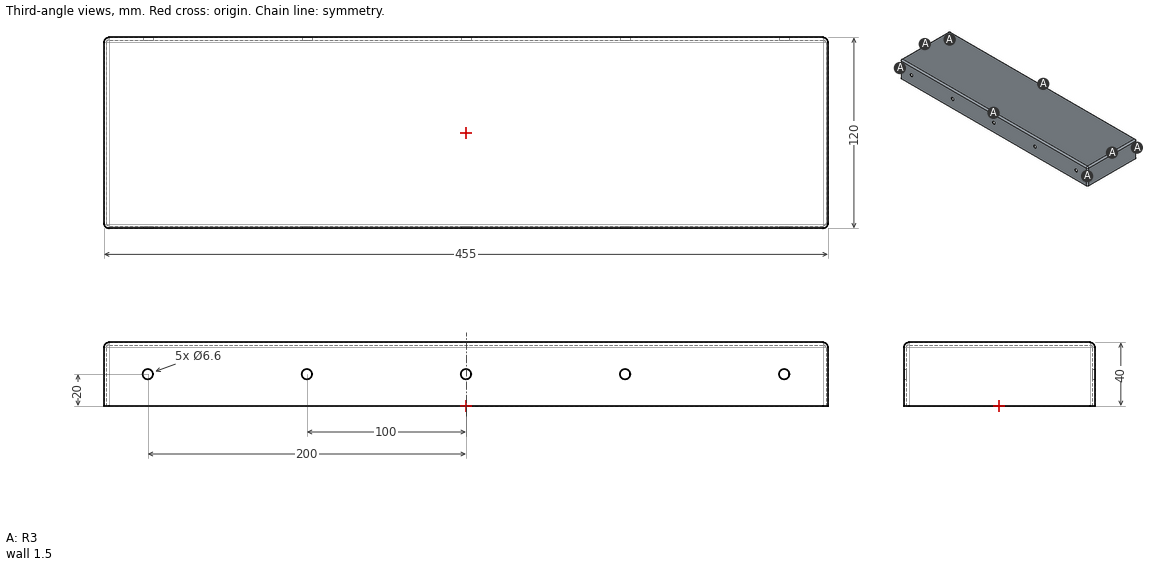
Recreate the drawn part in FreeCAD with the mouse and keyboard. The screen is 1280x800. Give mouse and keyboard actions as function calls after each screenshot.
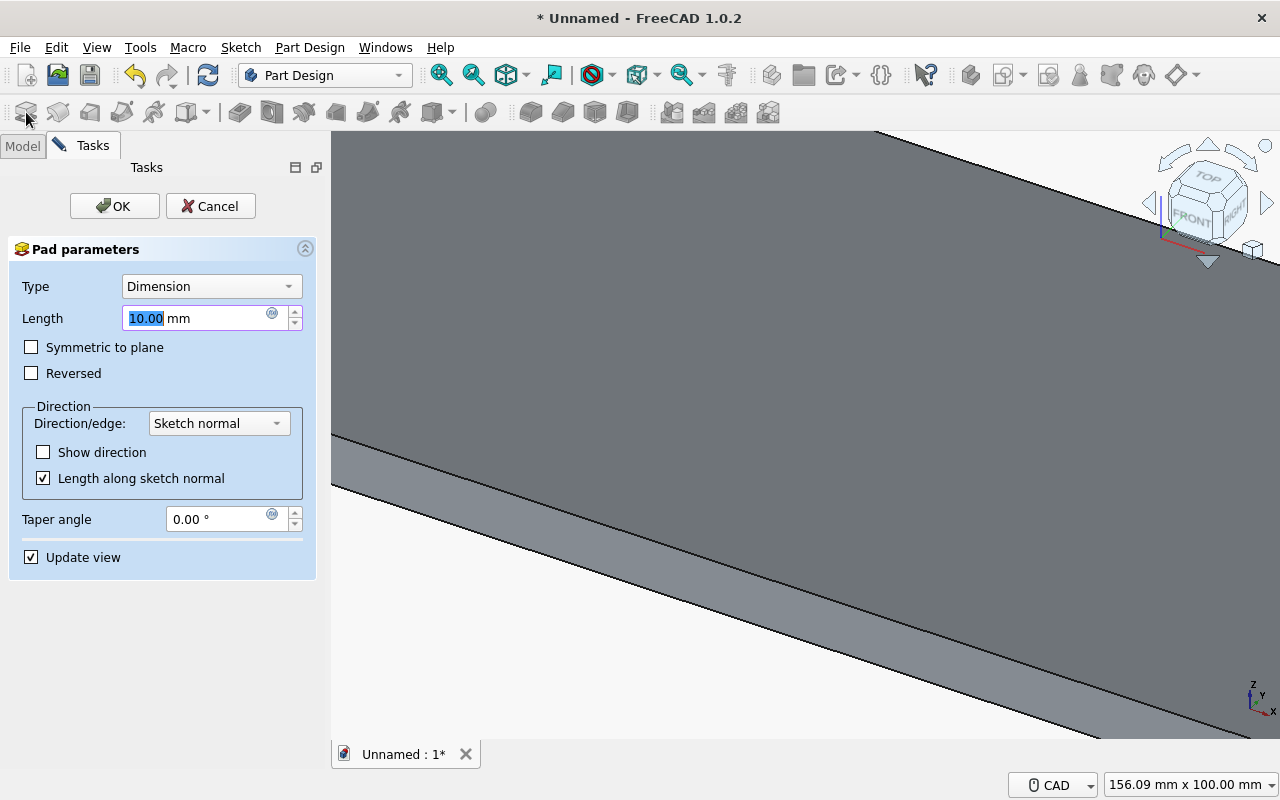
text(40)
key(Tab)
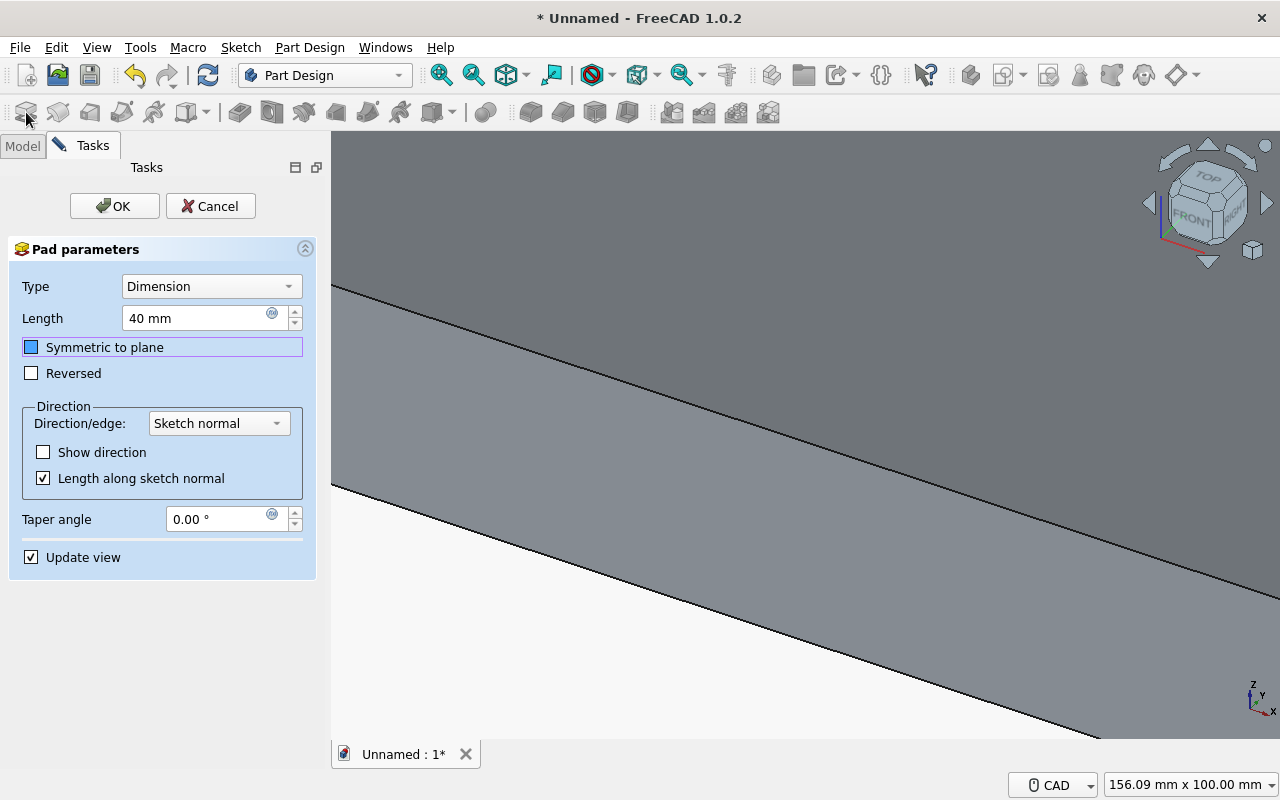
click(115, 206)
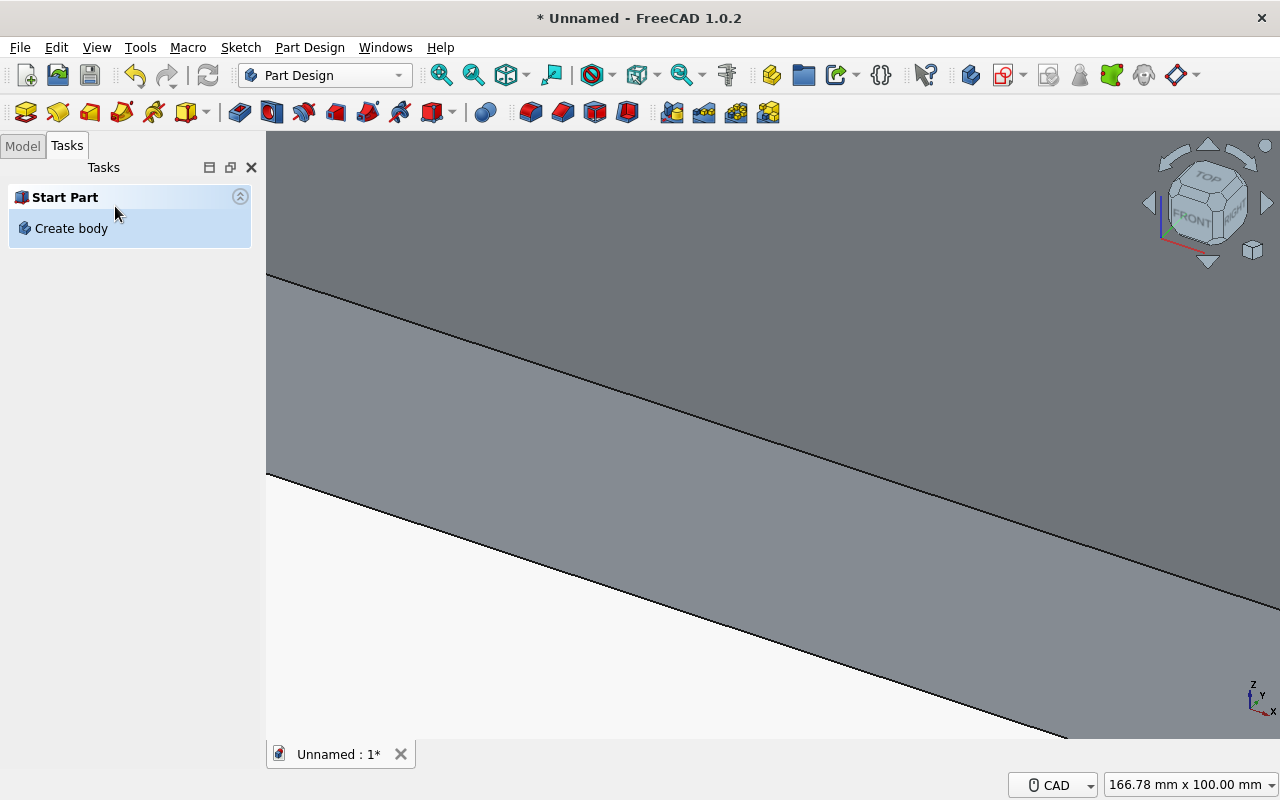
key(v)
key(f)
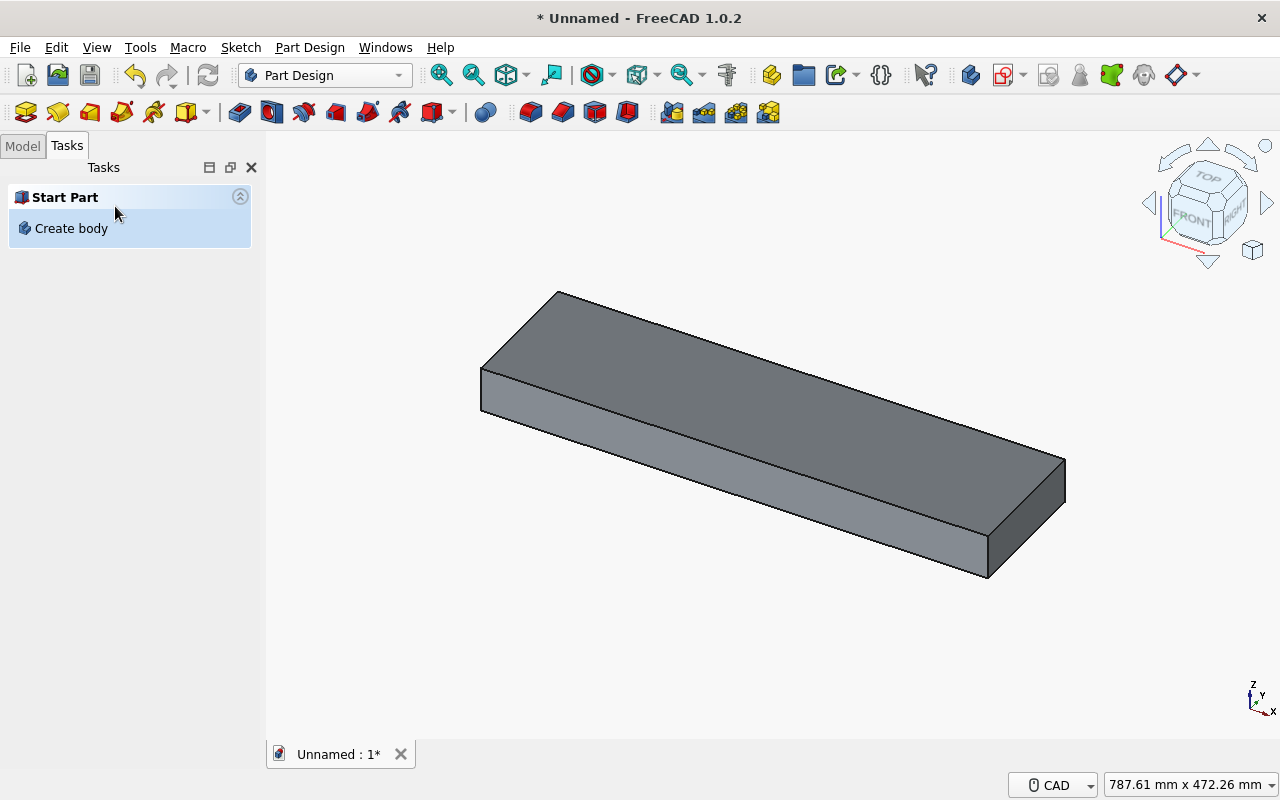
click(918, 461)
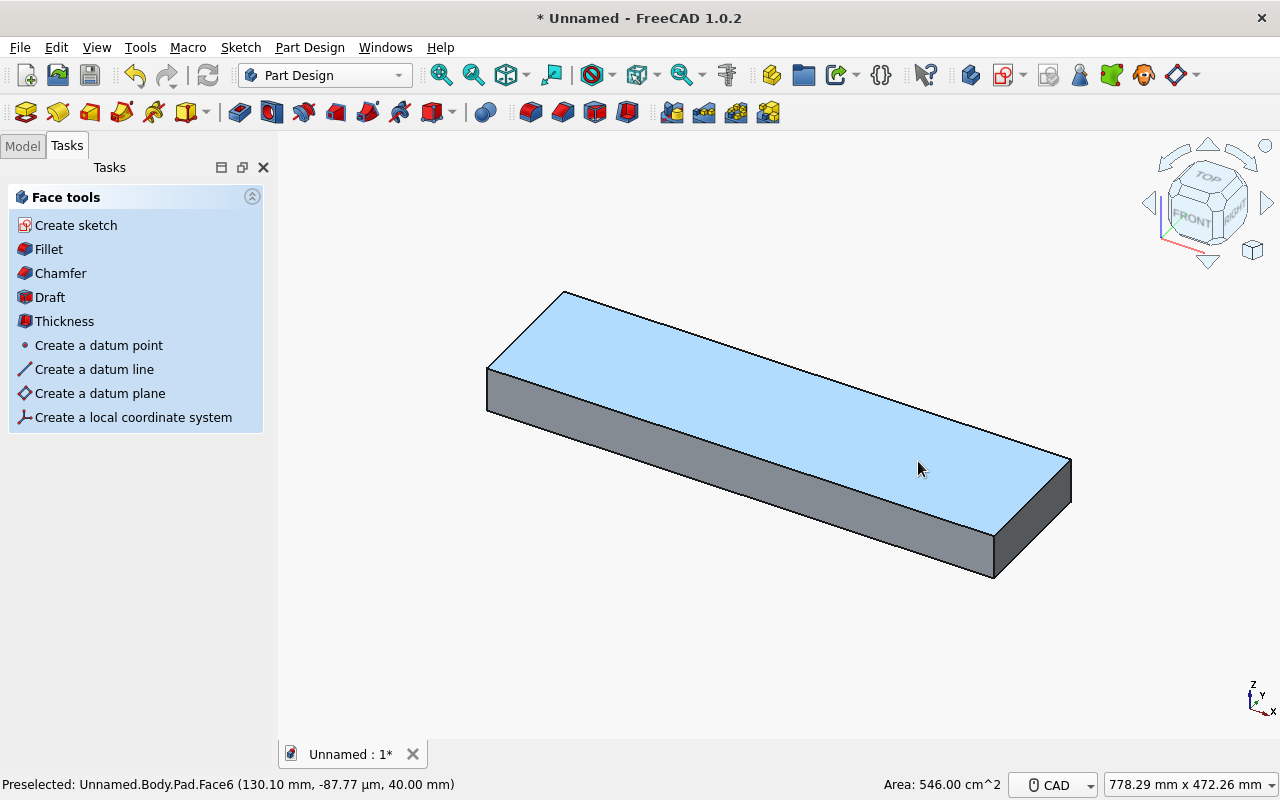
click(994, 556, ctrl)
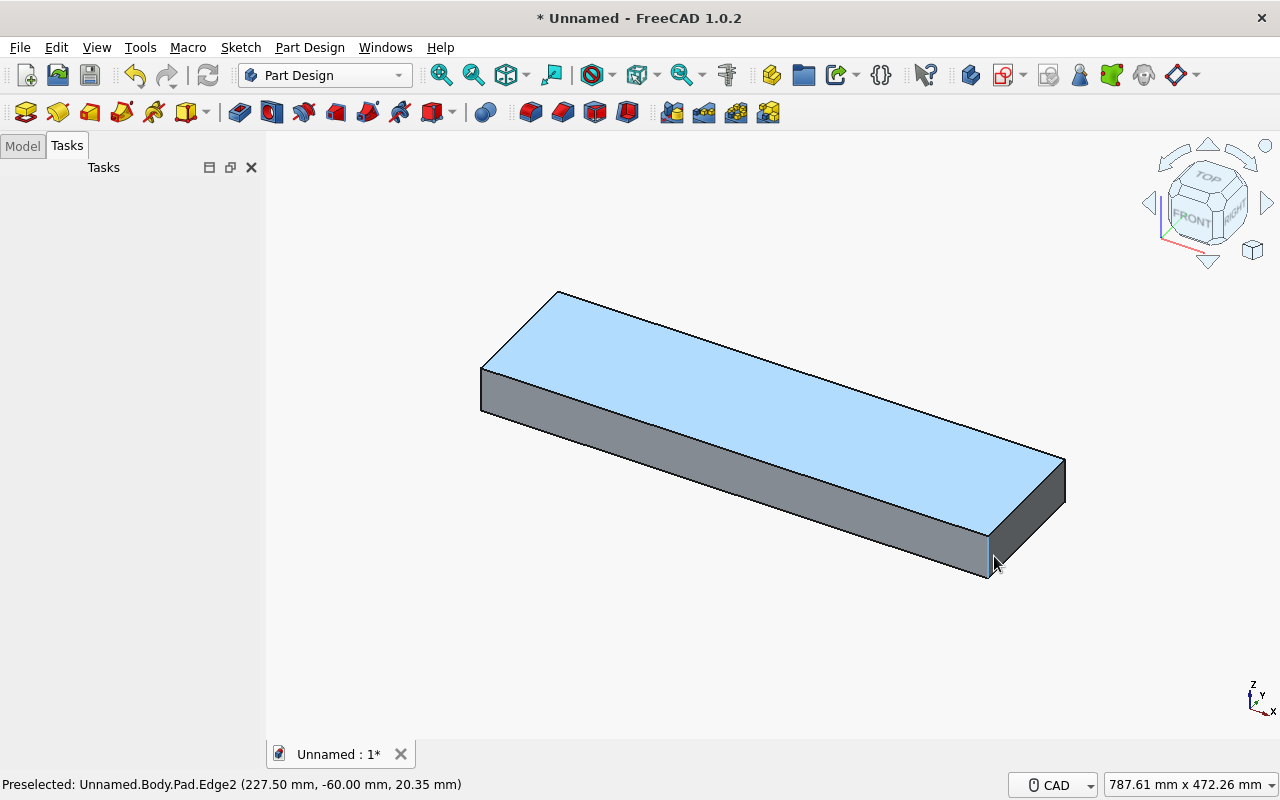
key(0)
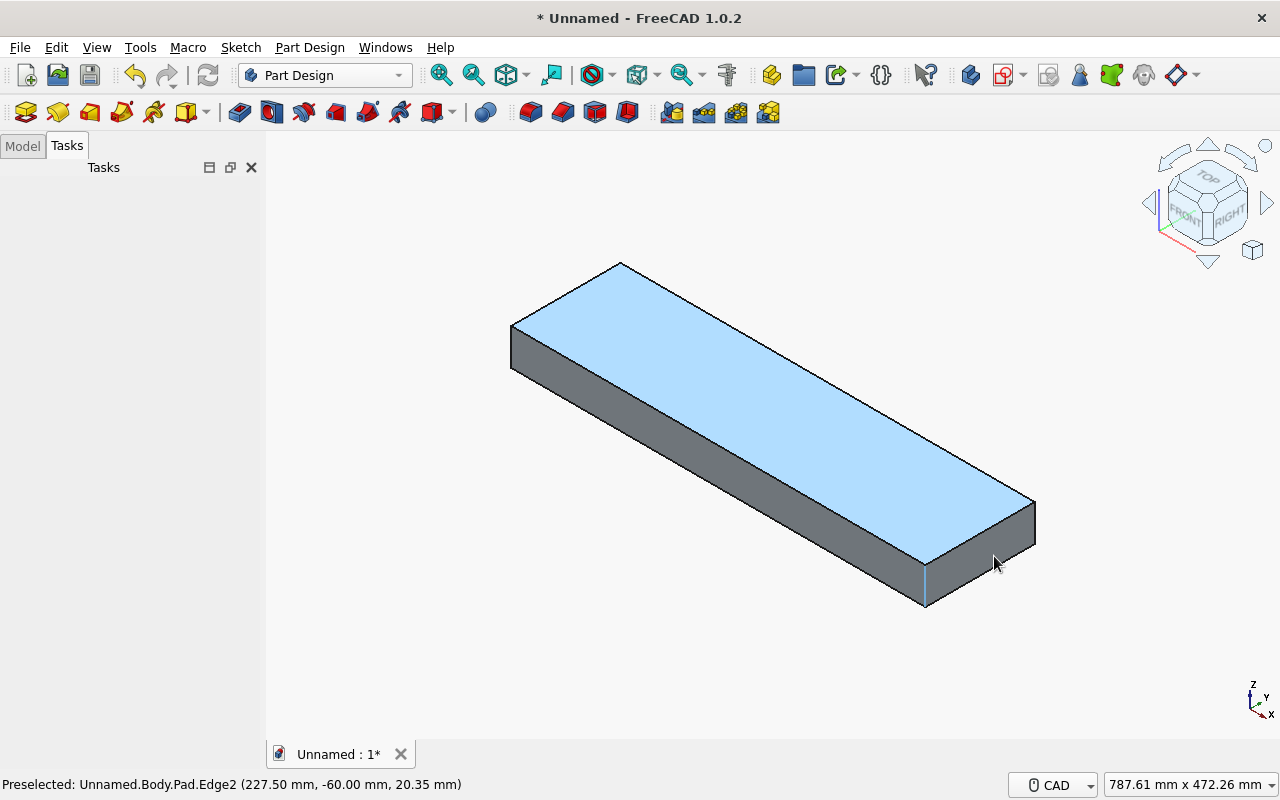
key(2)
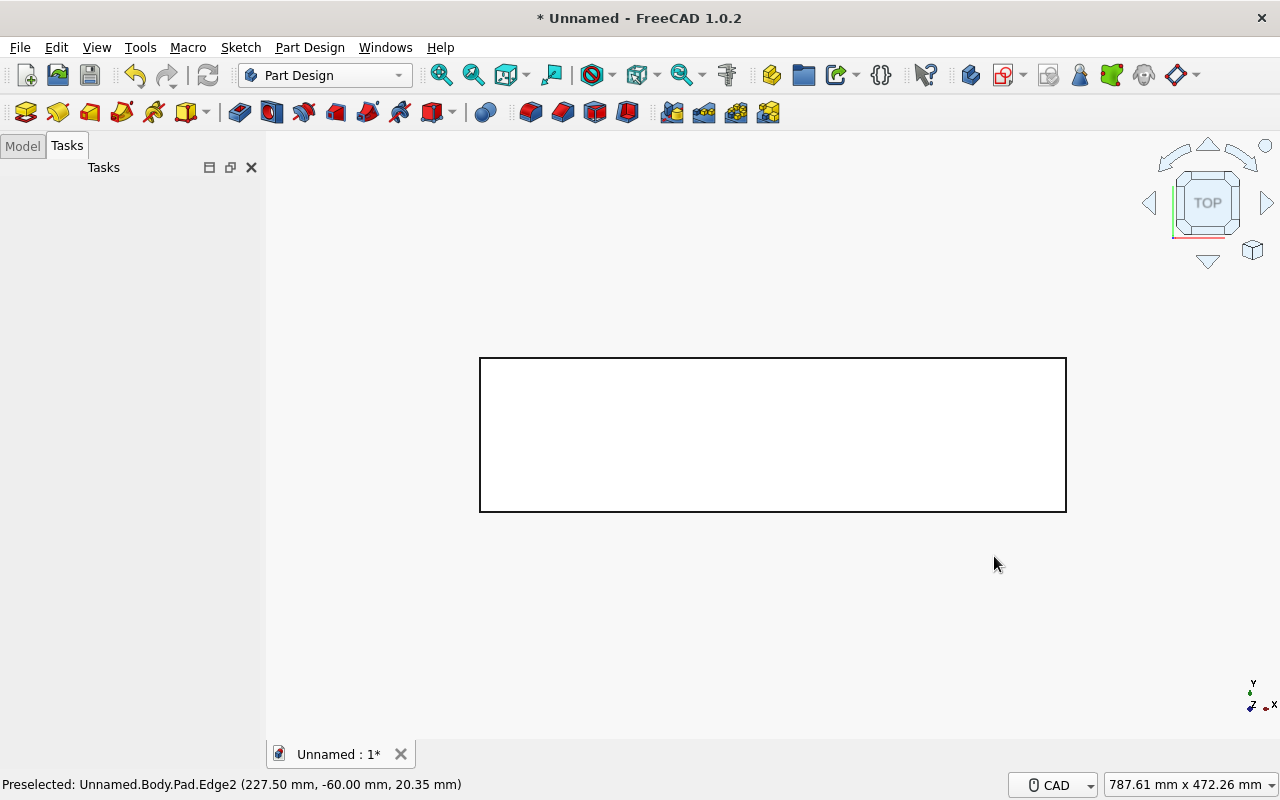
key(1)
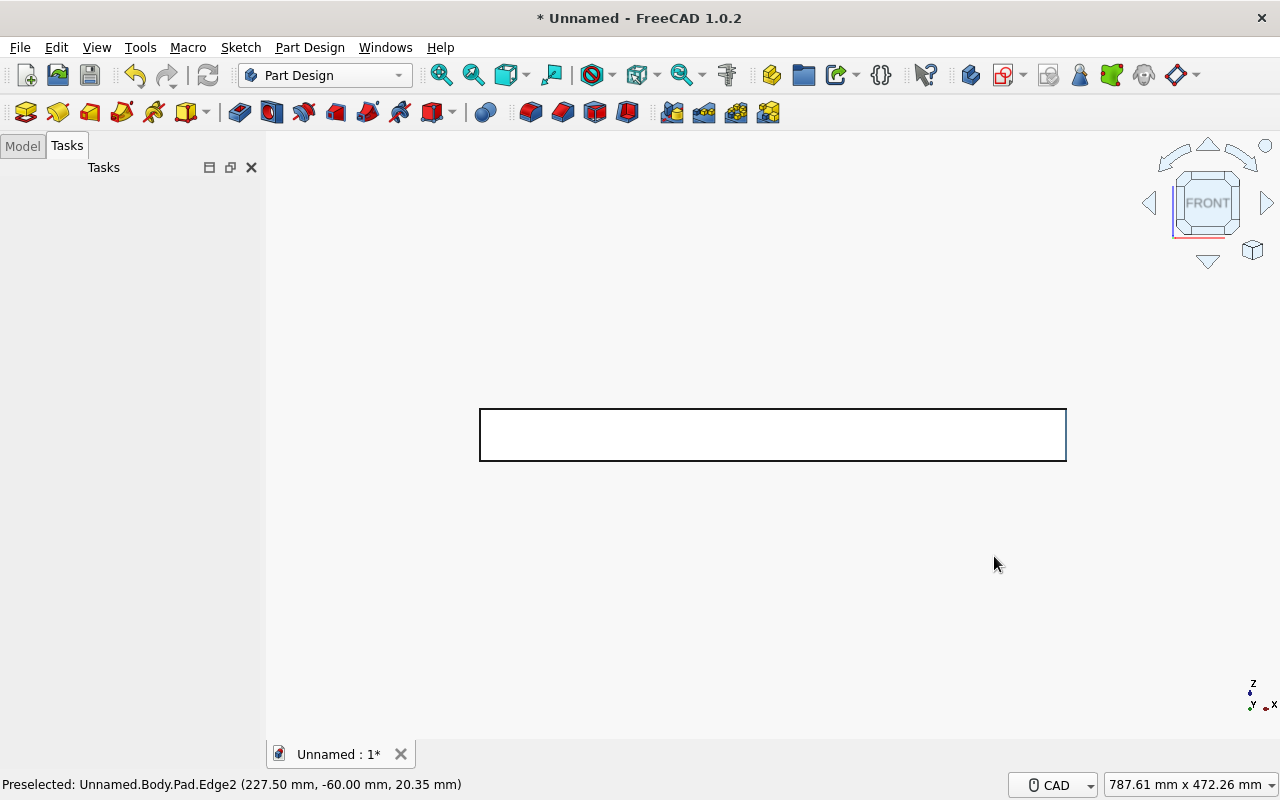
click(480, 434, ctrl)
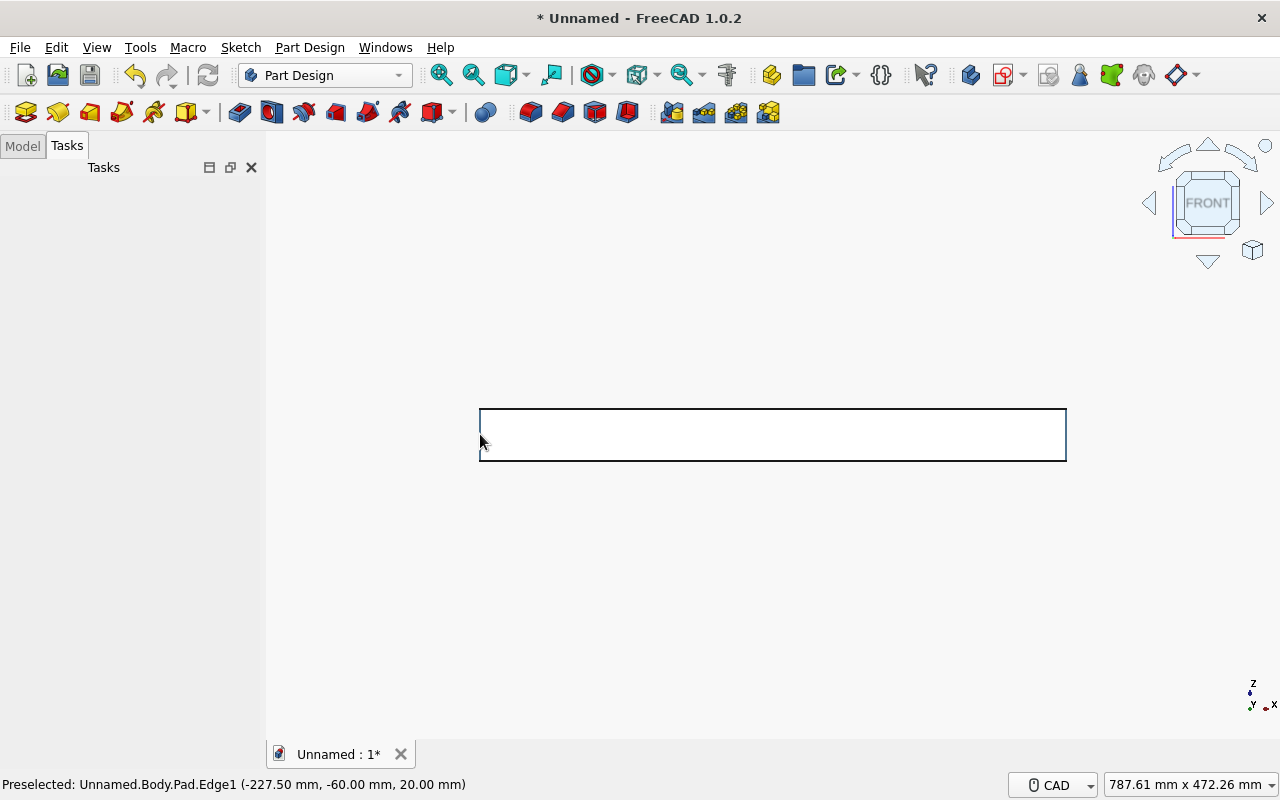
key(3)